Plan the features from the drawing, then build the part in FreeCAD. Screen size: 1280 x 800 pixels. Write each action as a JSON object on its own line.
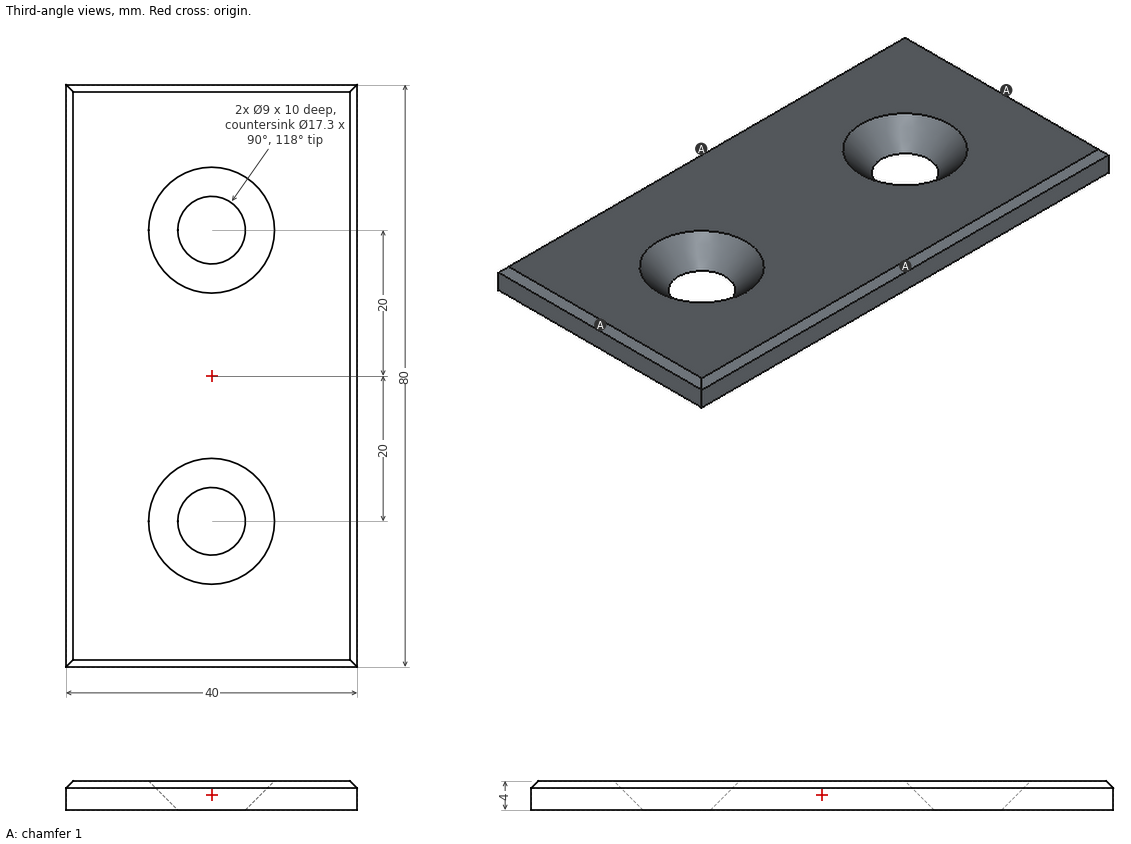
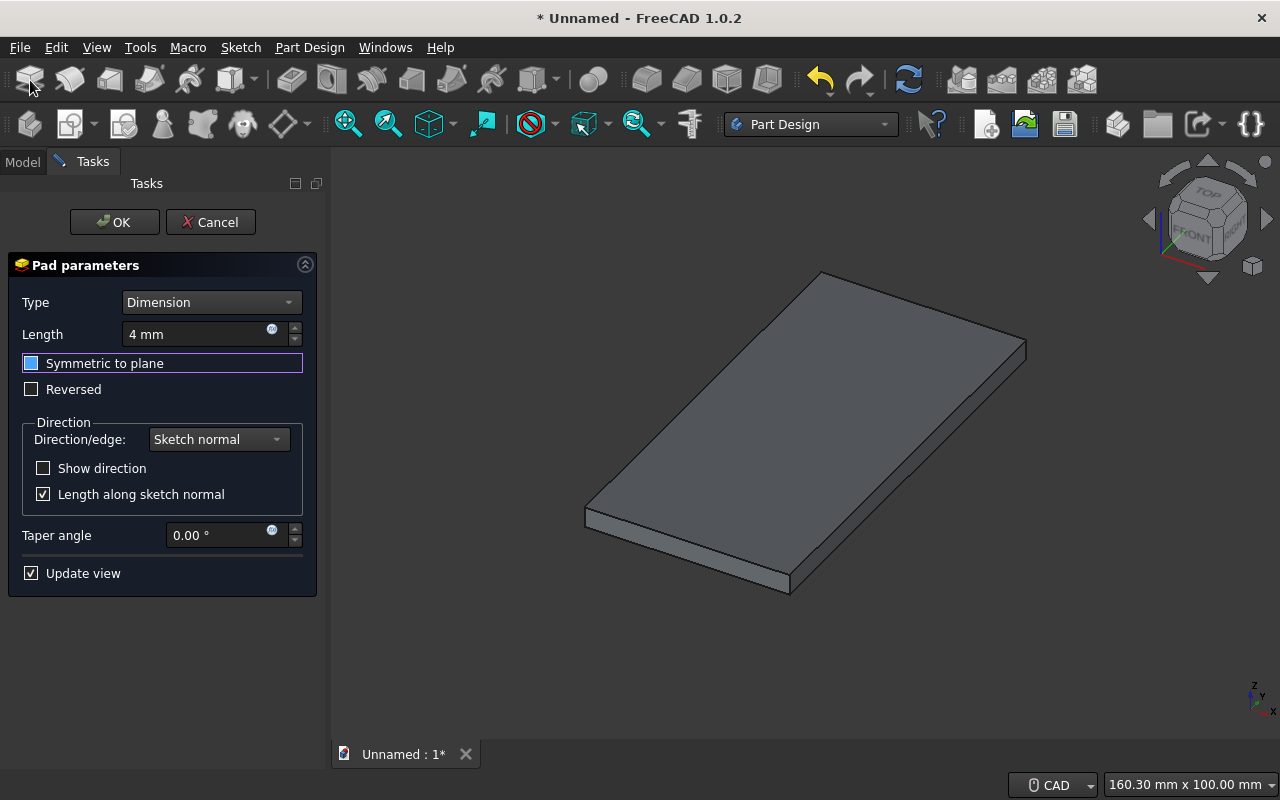
{"action": "left_click", "coordinate": [30, 363]}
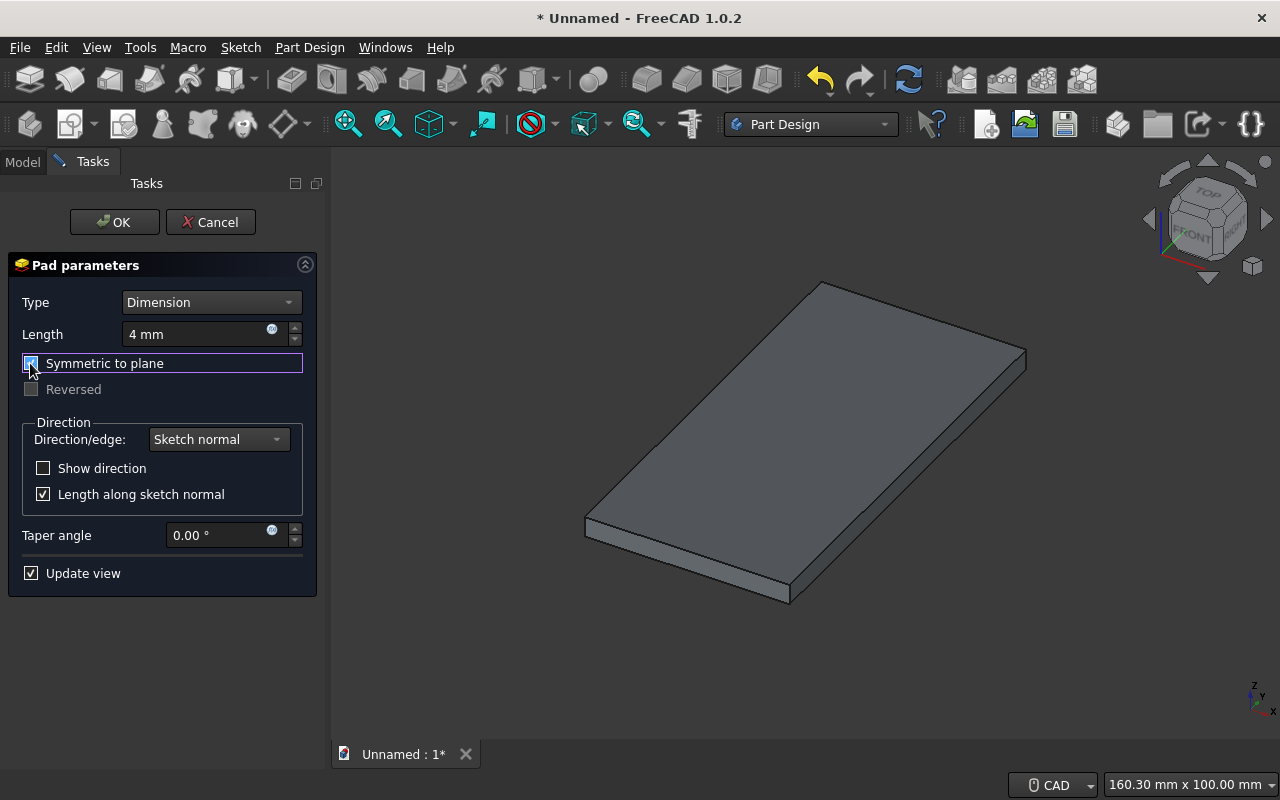
{"action": "left_click", "coordinate": [115, 222]}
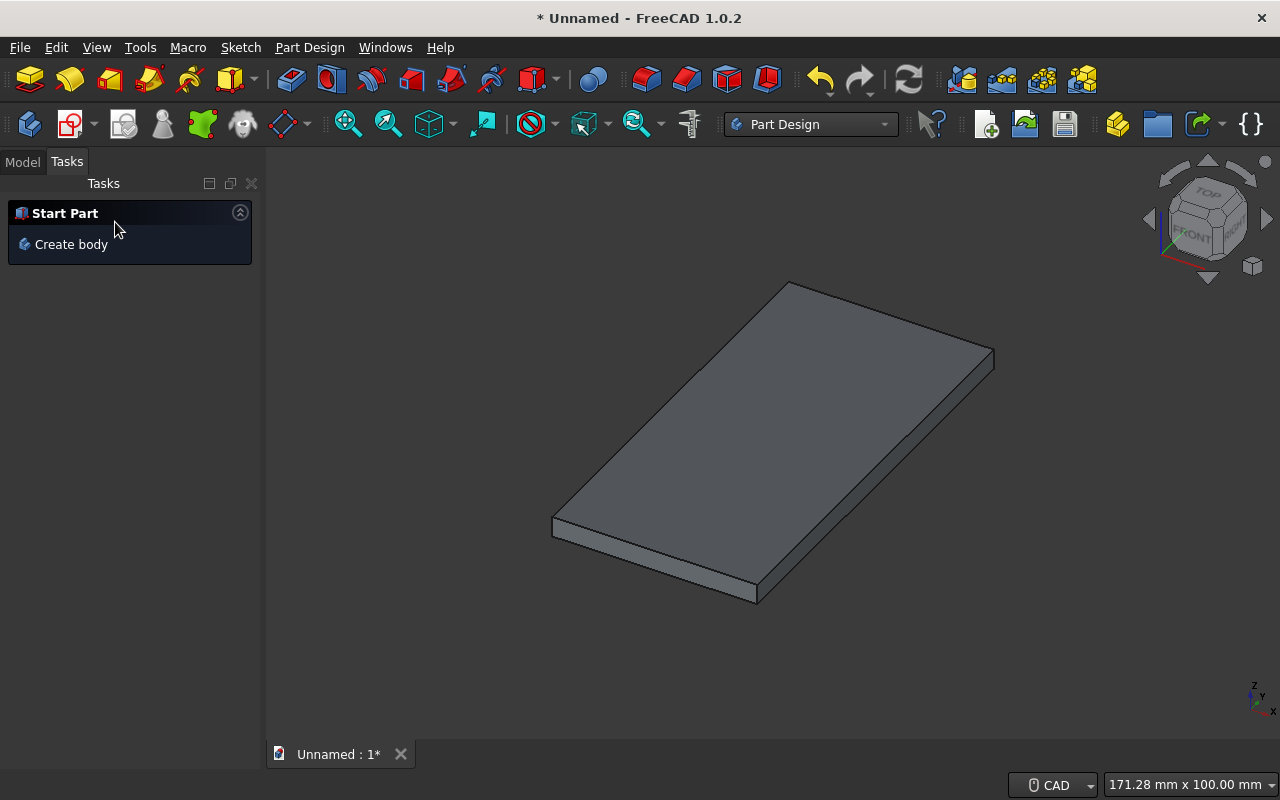
{"action": "left_click", "coordinate": [807, 399]}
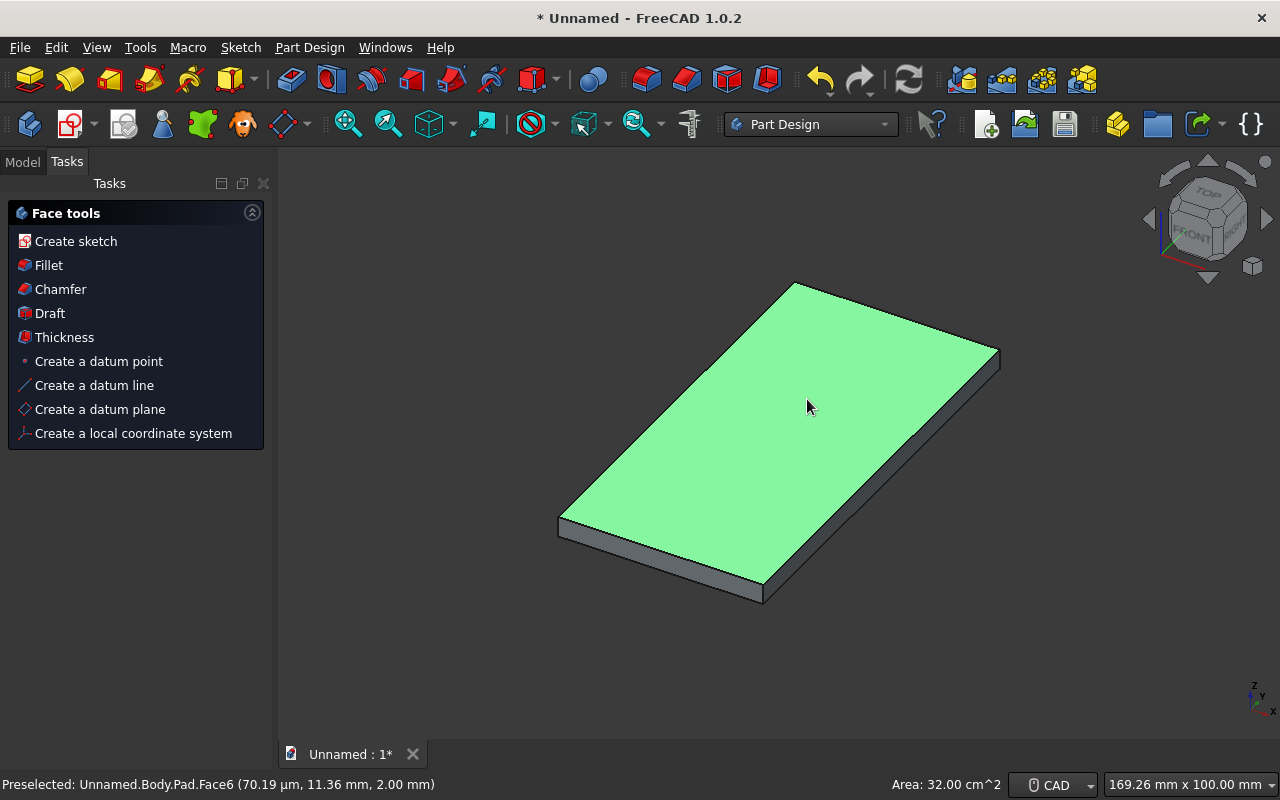
{"action": "left_click", "coordinate": [70, 124]}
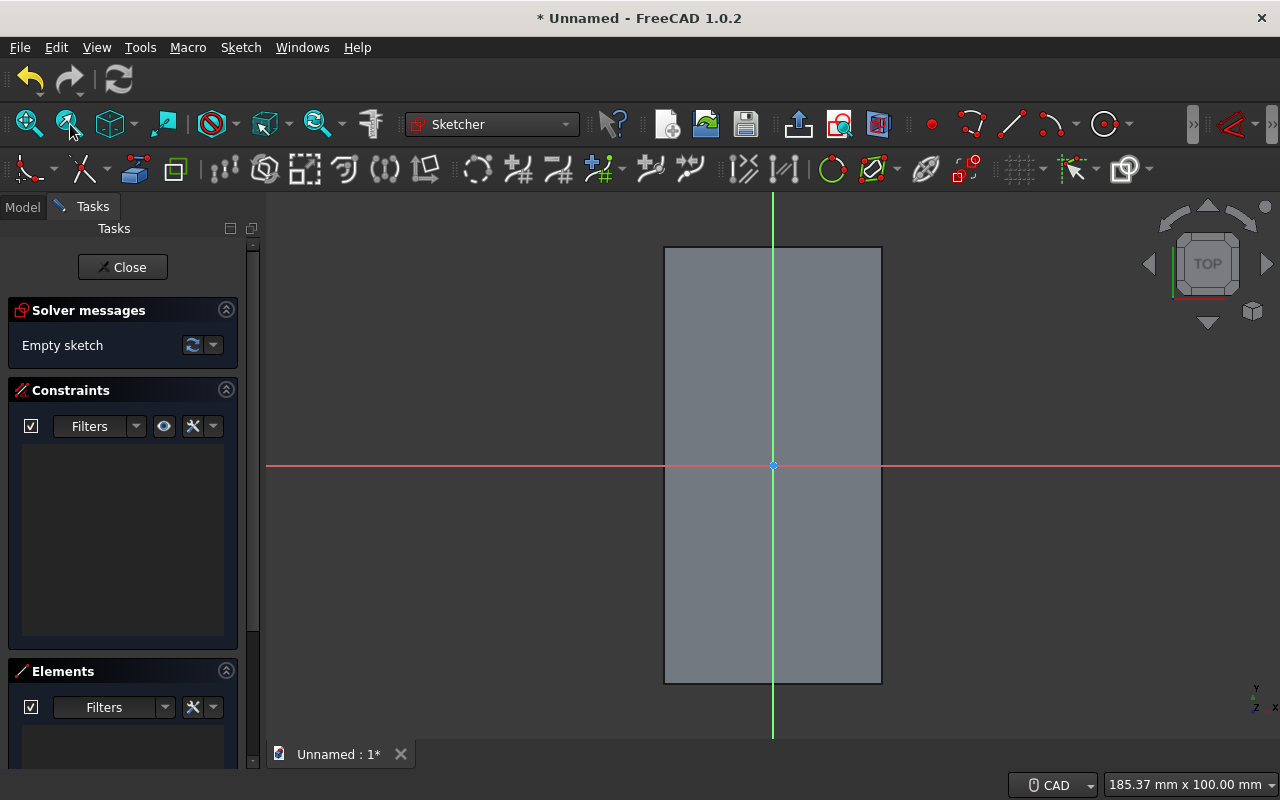
{"action": "key", "text": "g c"}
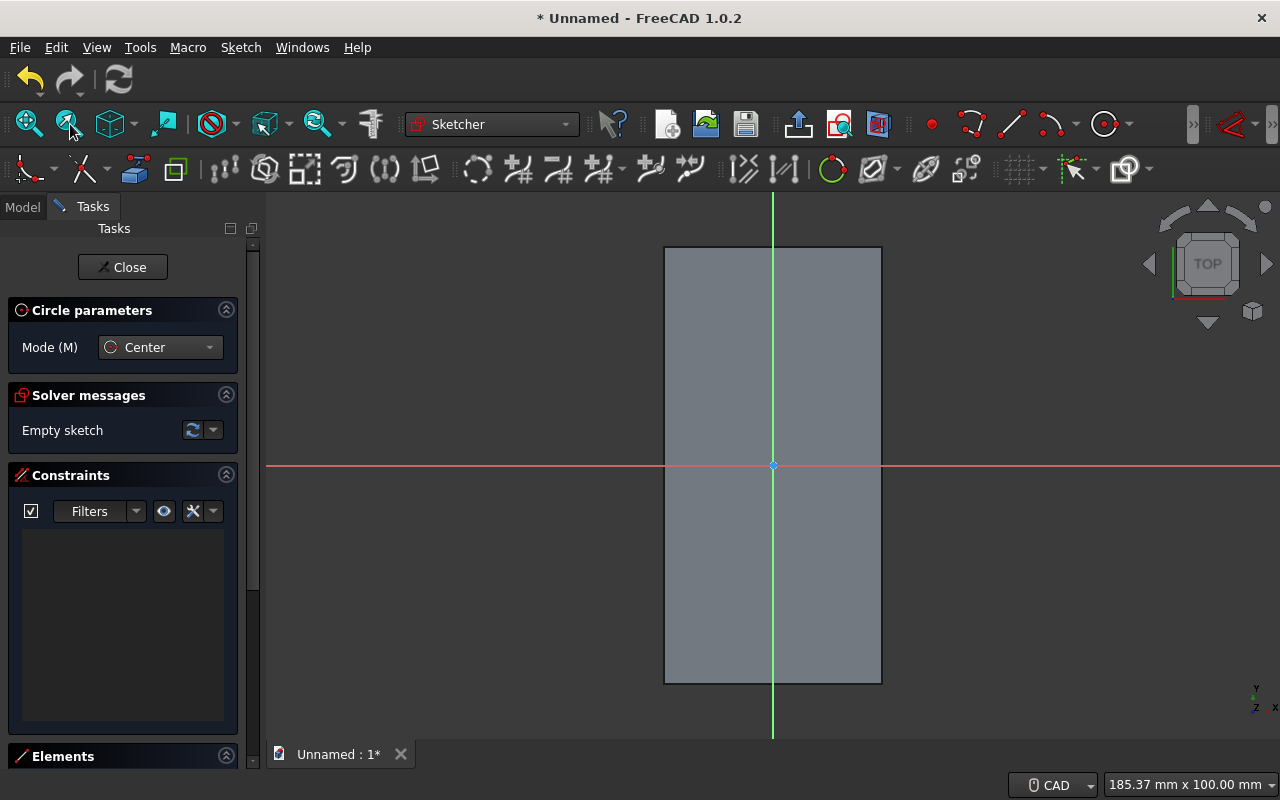
{"action": "left_click", "coordinate": [773, 356]}
{"action": "mouse_move", "coordinate": [790, 339]}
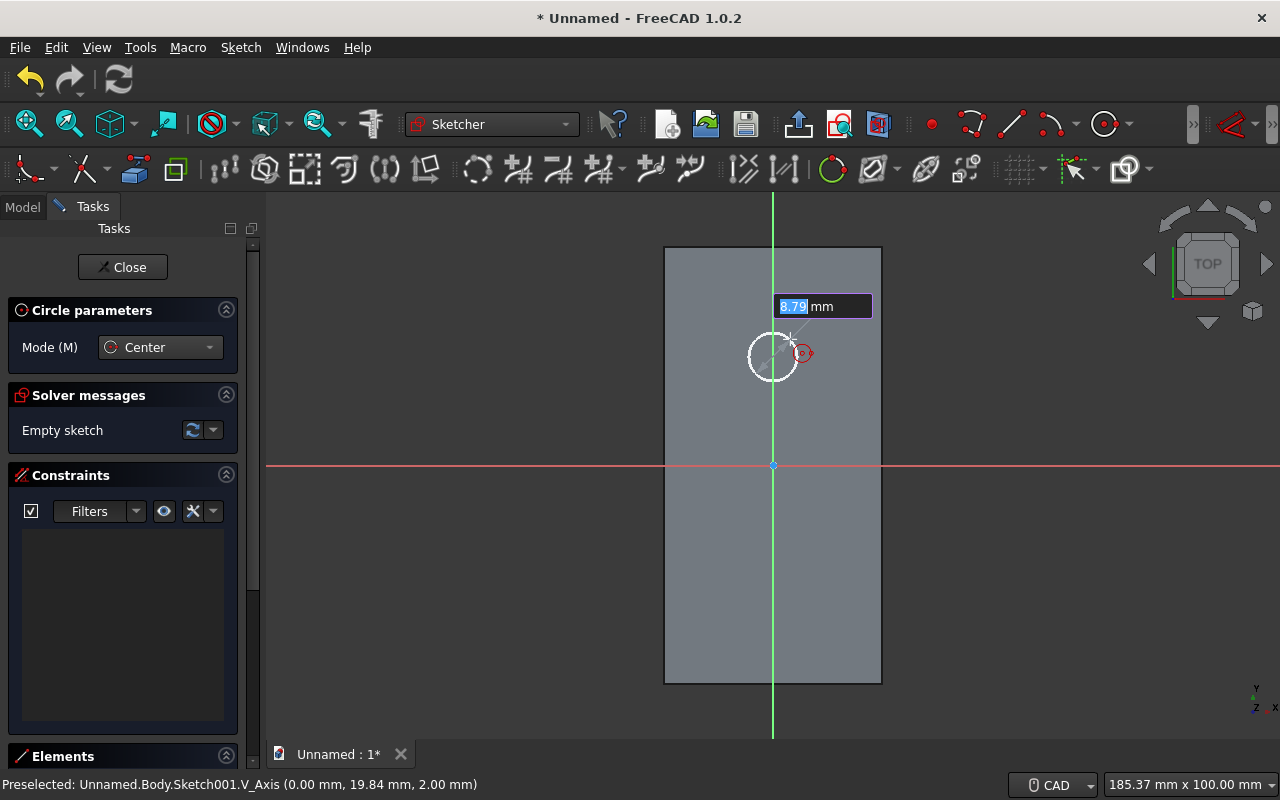
{"action": "type", "text": "9"}
{"action": "key", "text": "Return"}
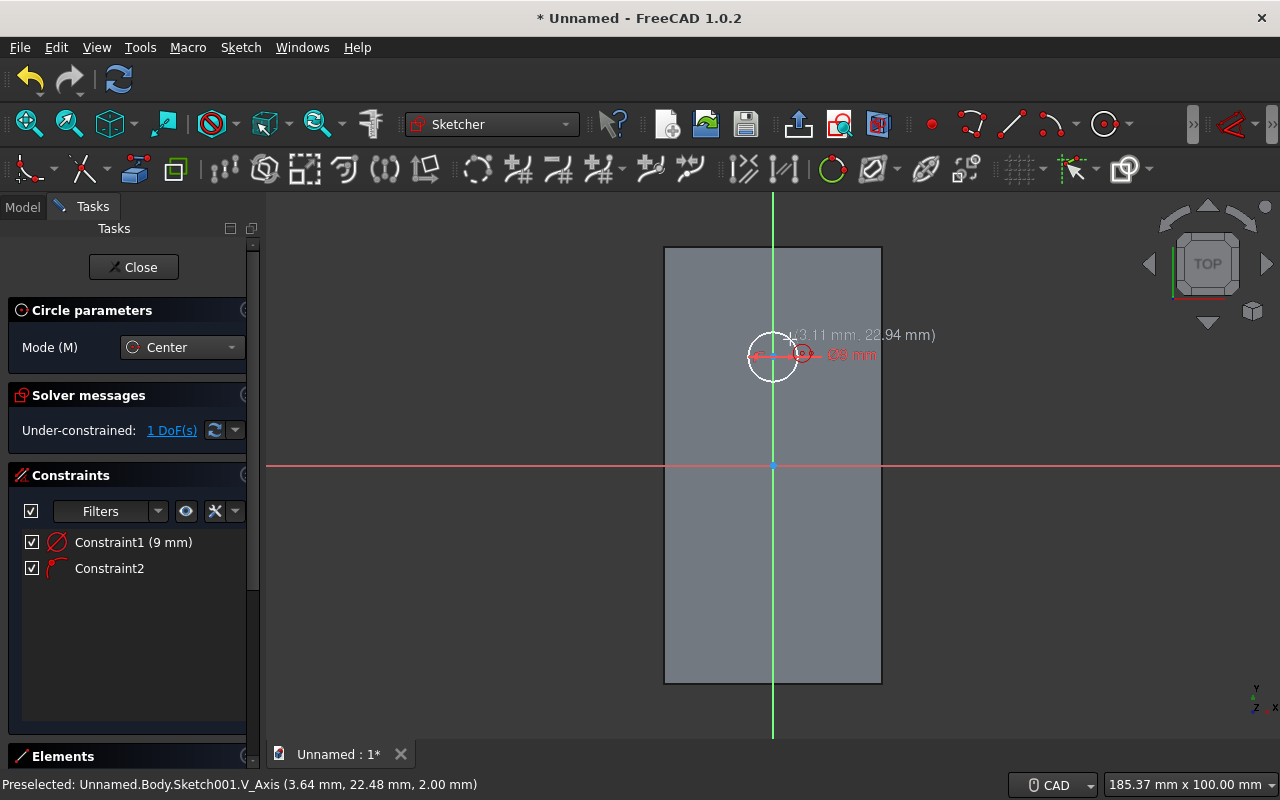
{"action": "left_click", "coordinate": [773, 575]}
{"action": "mouse_move", "coordinate": [790, 557]}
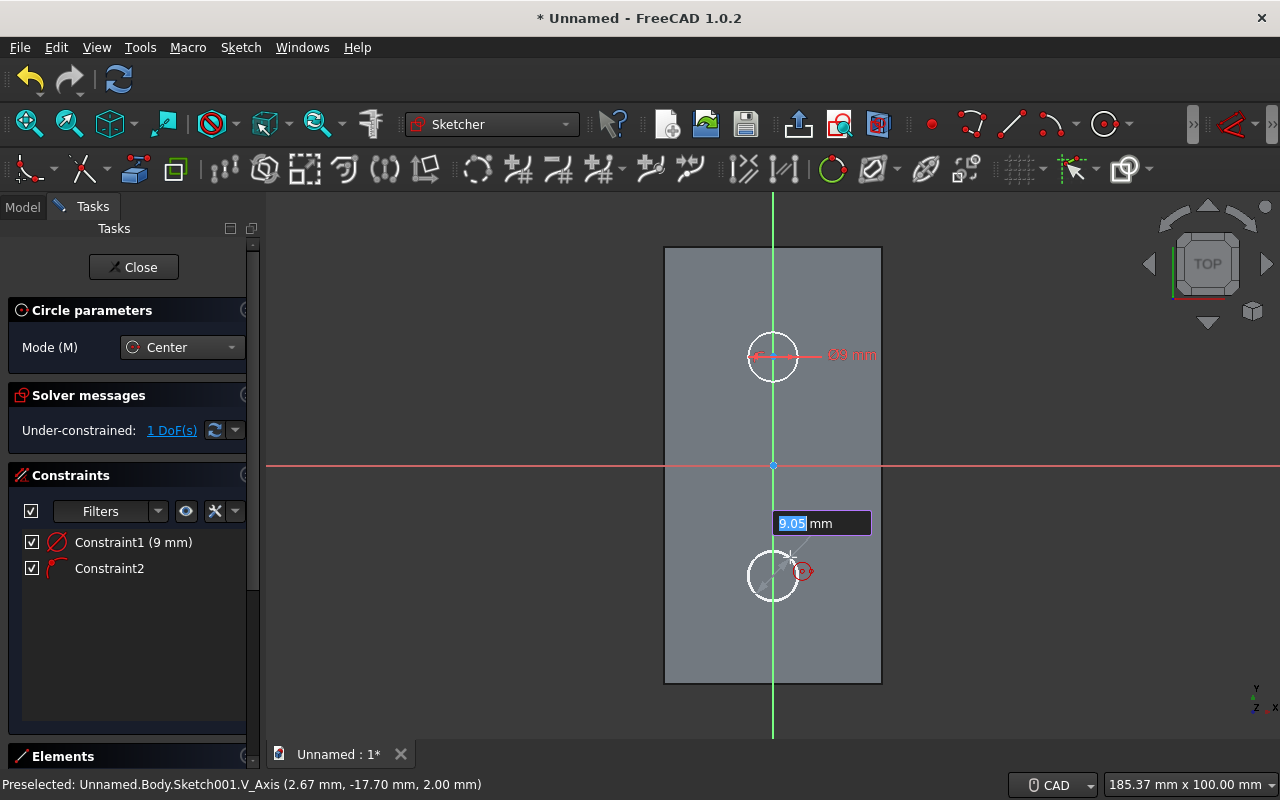
{"action": "type", "text": "9"}
{"action": "key", "text": "Return"}
{"action": "key", "text": "Escape"}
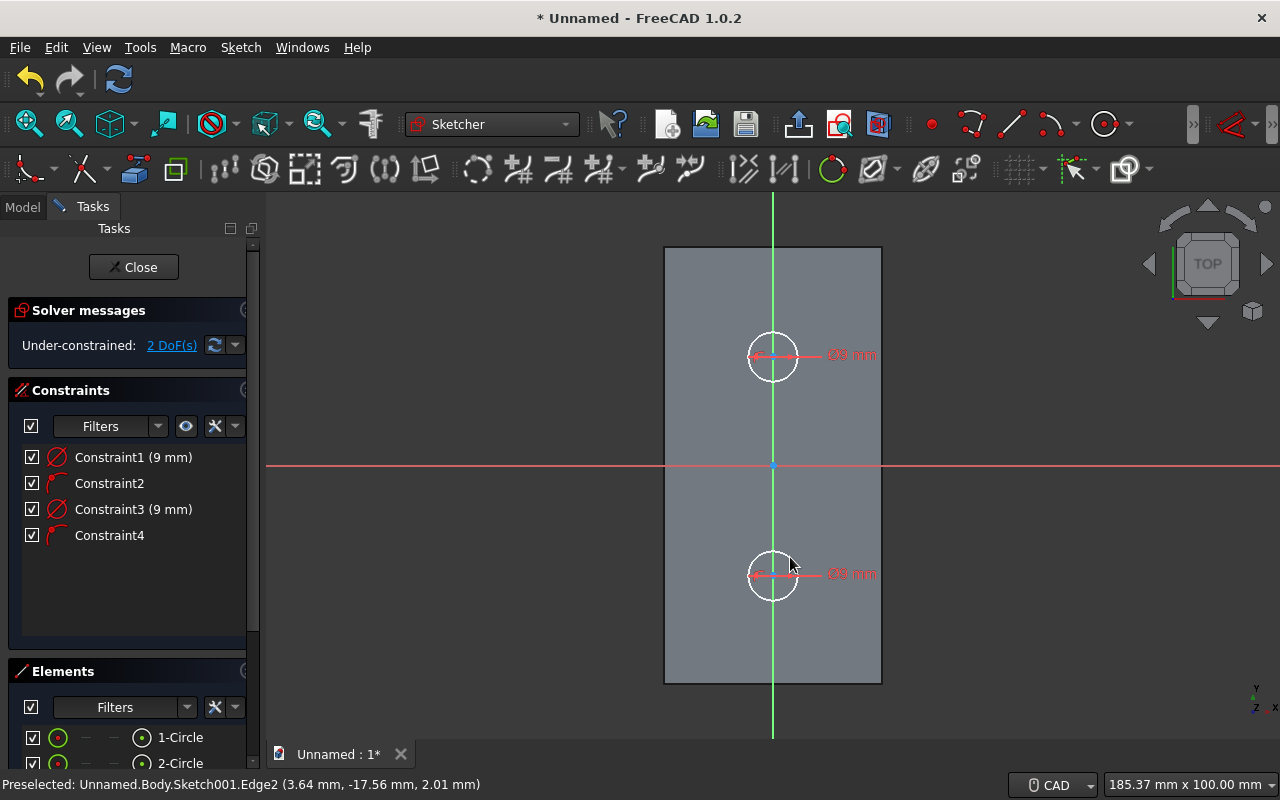
{"action": "key", "text": "d"}